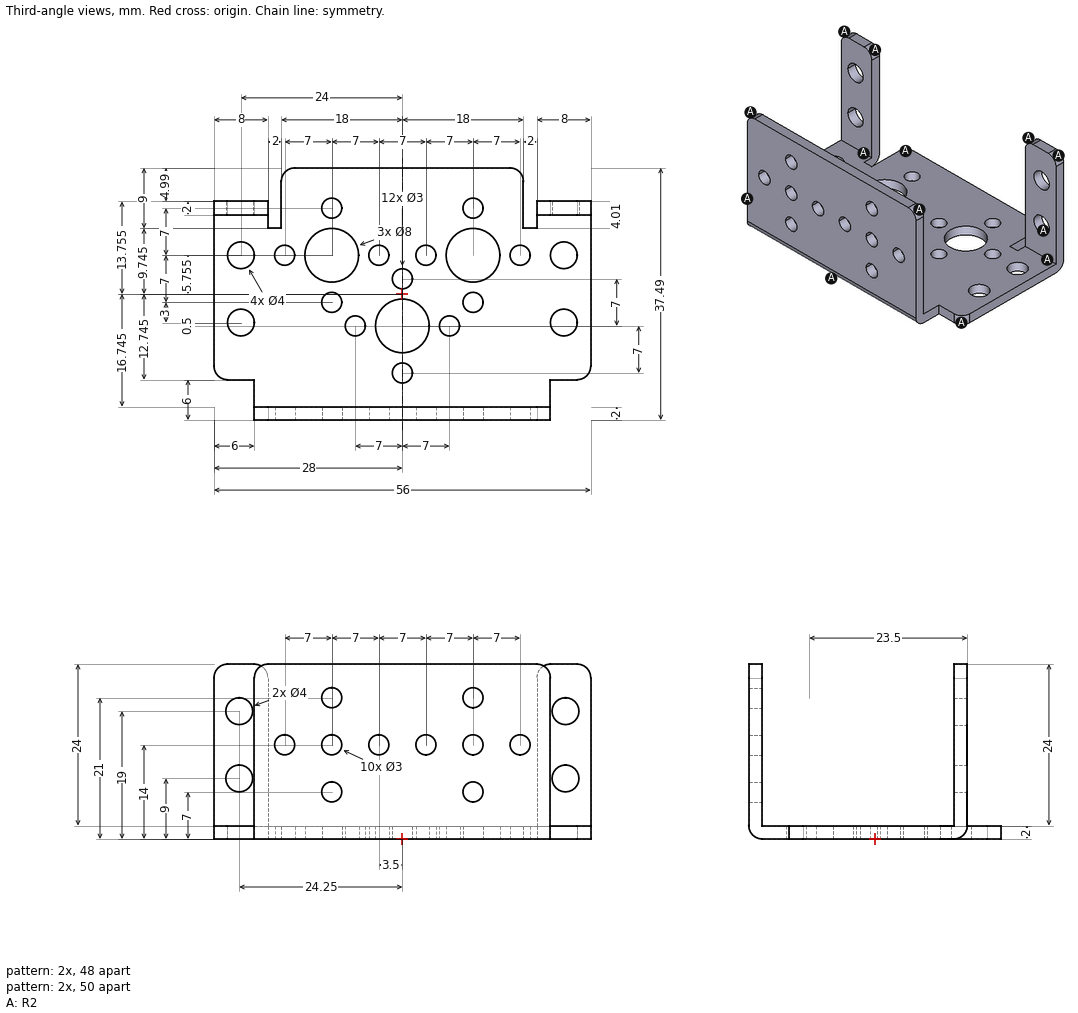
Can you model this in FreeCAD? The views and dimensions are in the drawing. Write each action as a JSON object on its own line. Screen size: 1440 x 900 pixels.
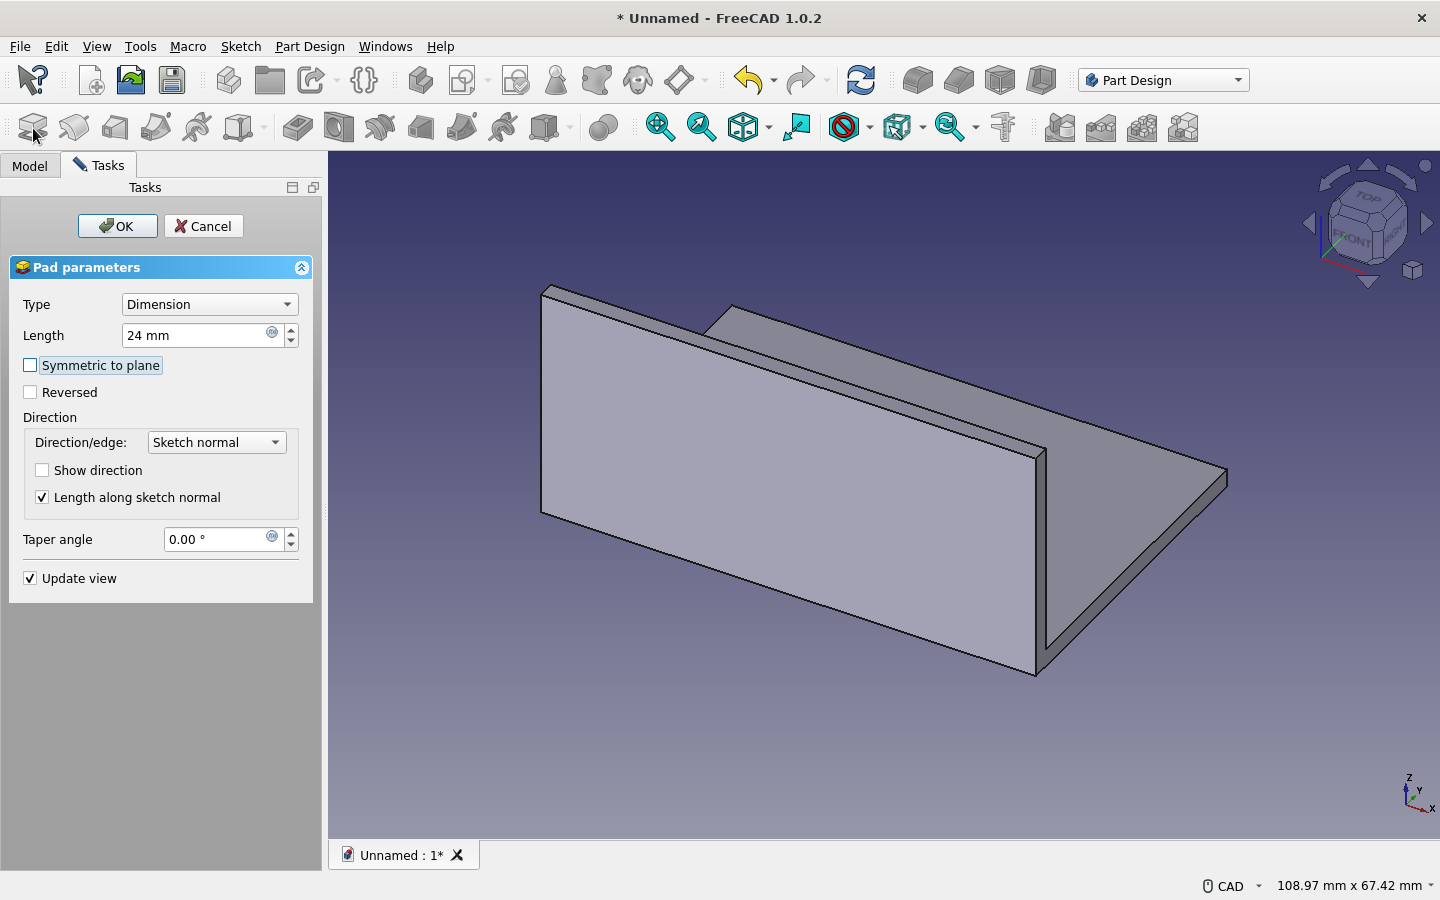
{"action": "left_click", "coordinate": [118, 226]}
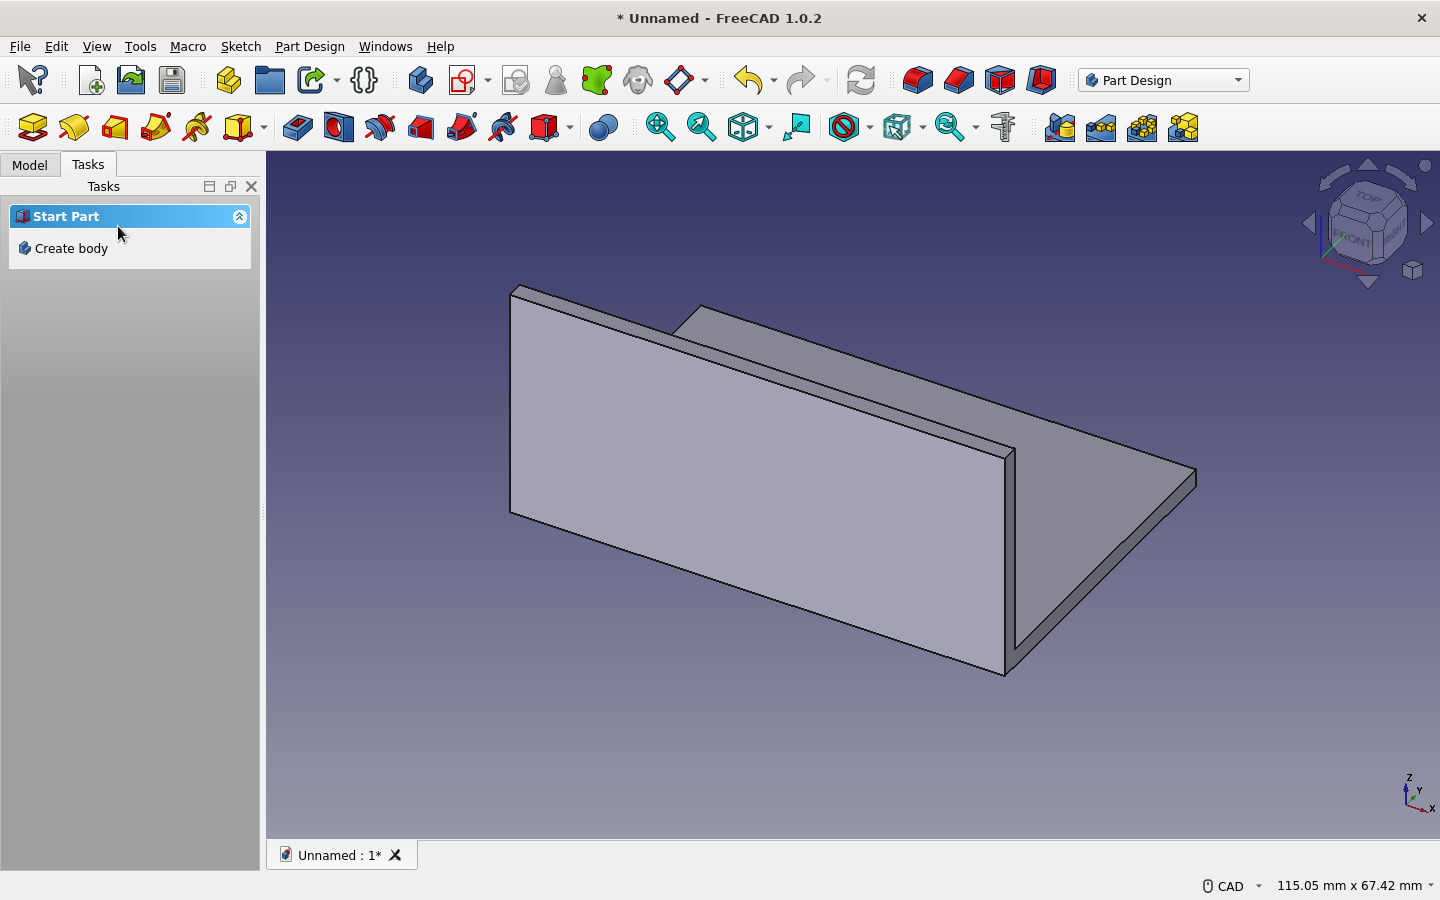
{"action": "key", "text": "v f"}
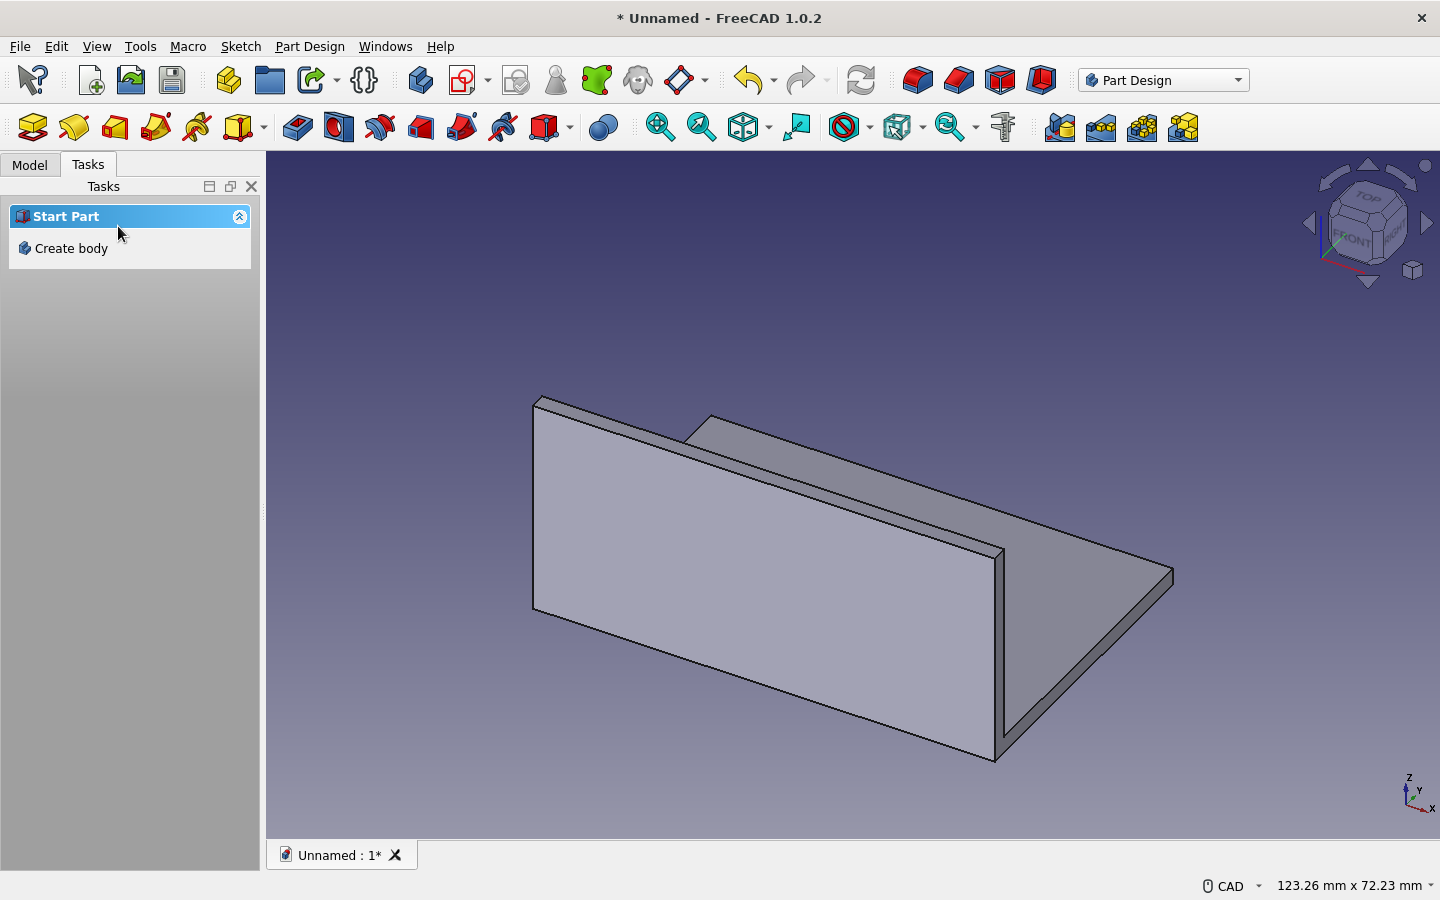
{"action": "key", "text": "0"}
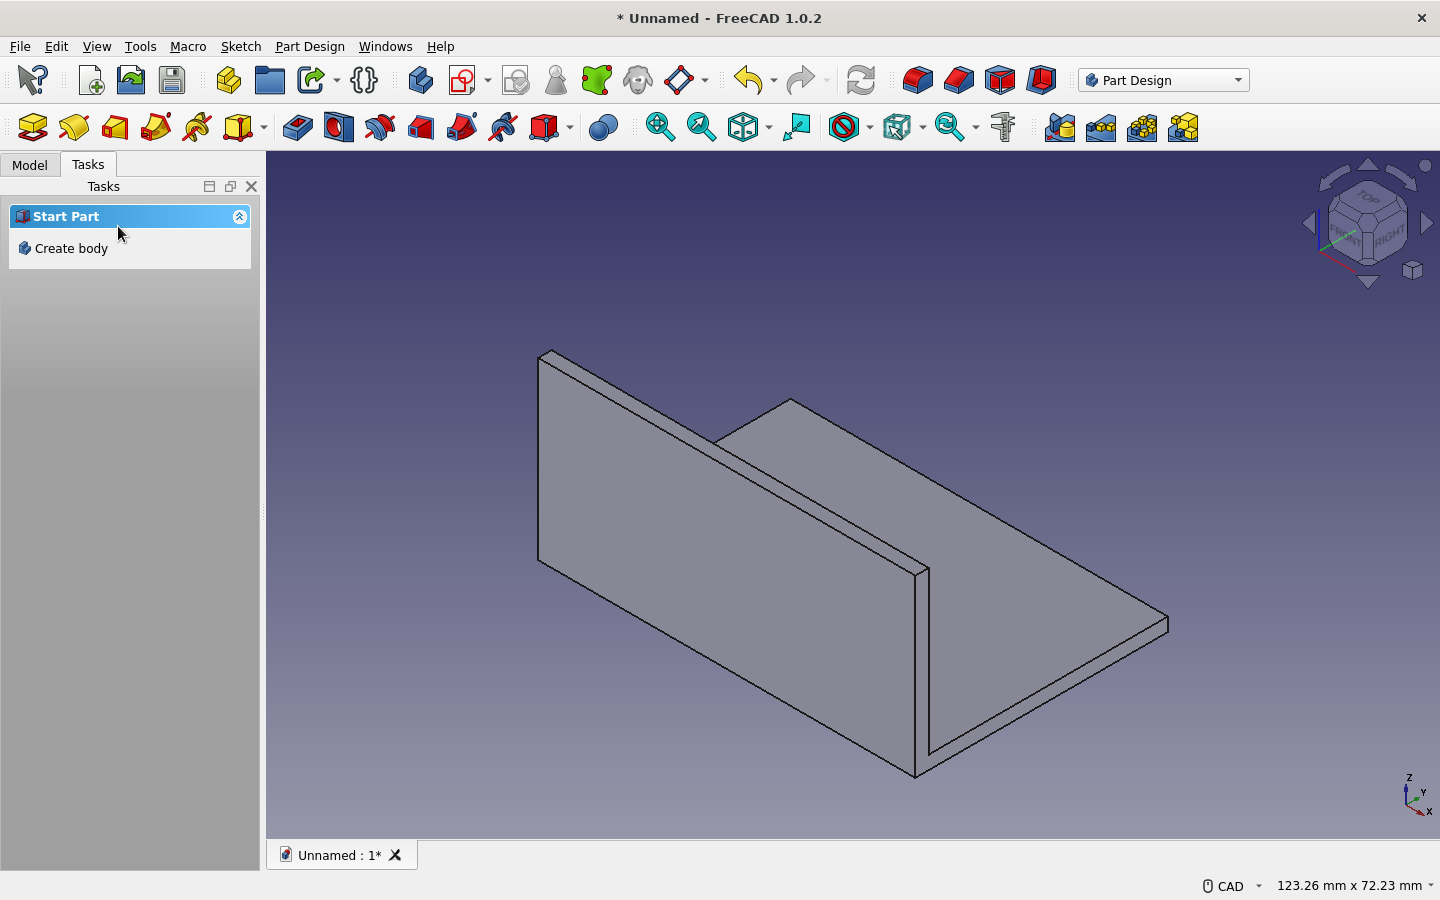
{"action": "left_click", "coordinate": [948, 587]}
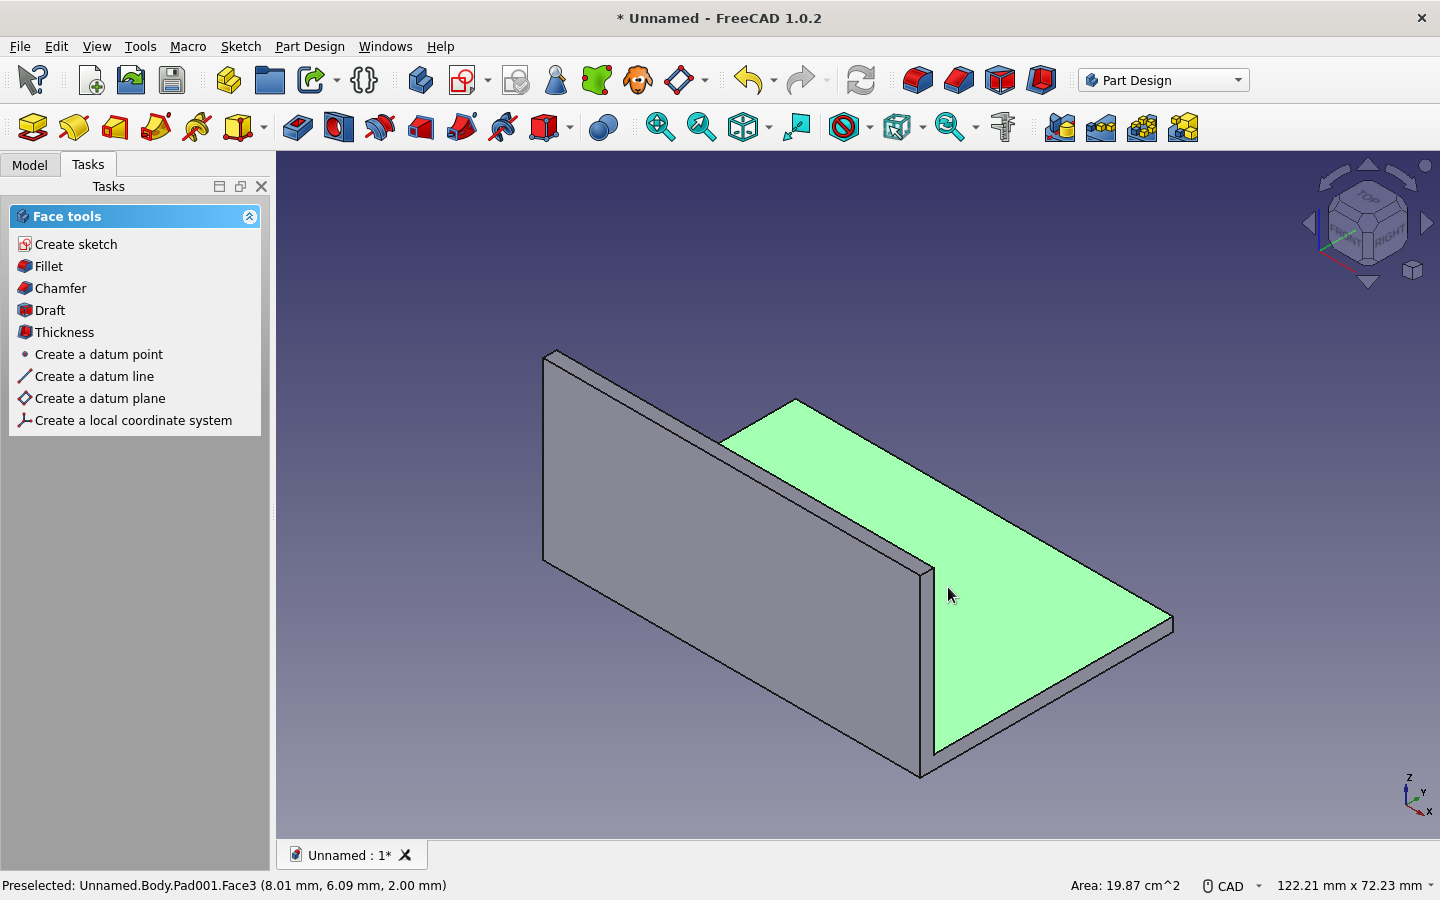
{"action": "left_click", "coordinate": [462, 80]}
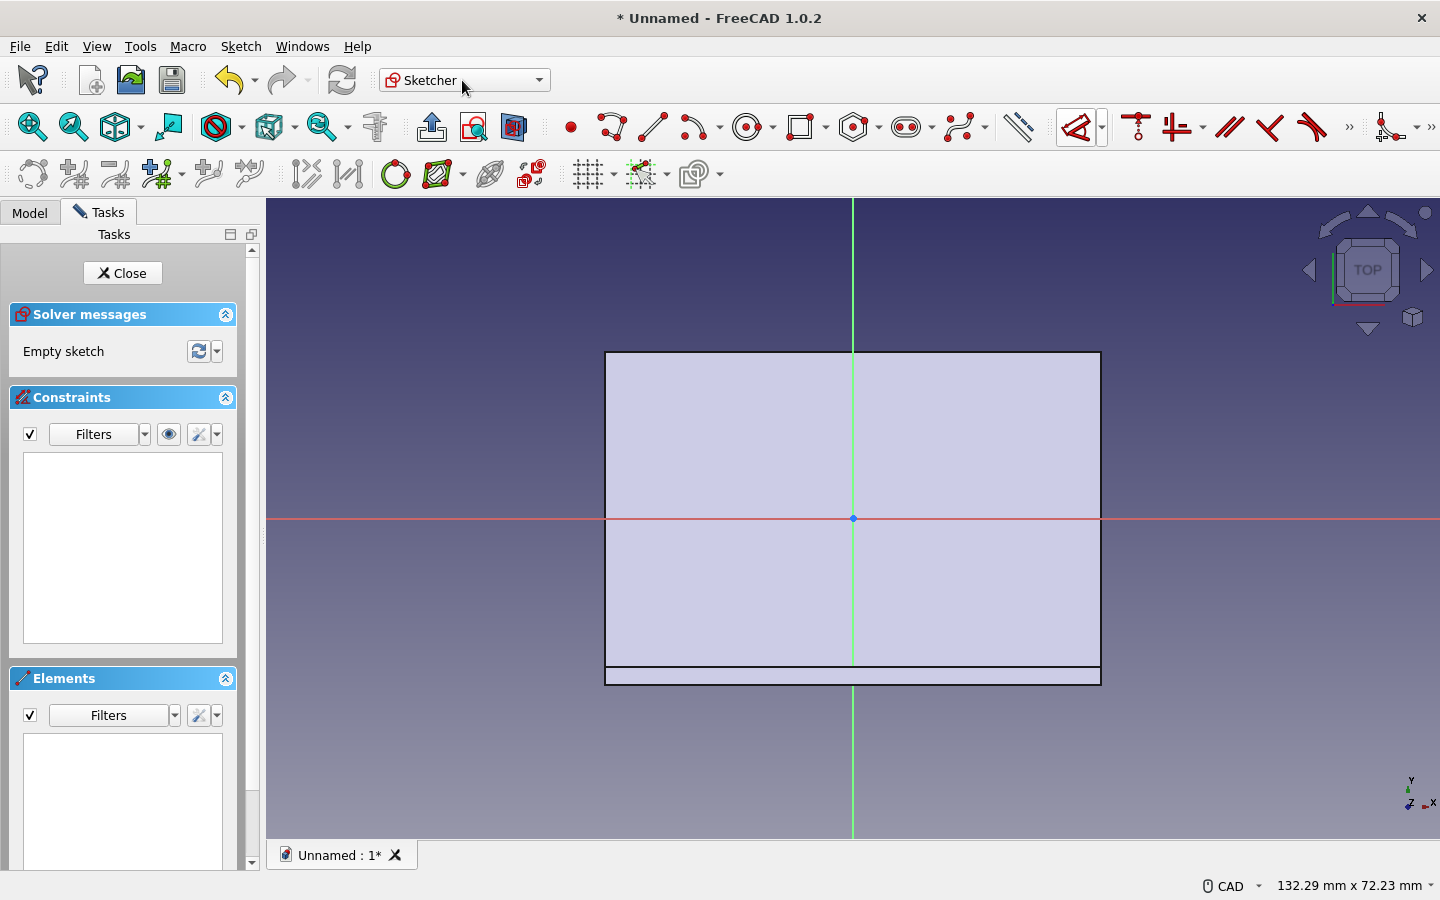
{"action": "scroll", "coordinate": [622, 391], "scroll_direction": "up", "scroll_amount": 11}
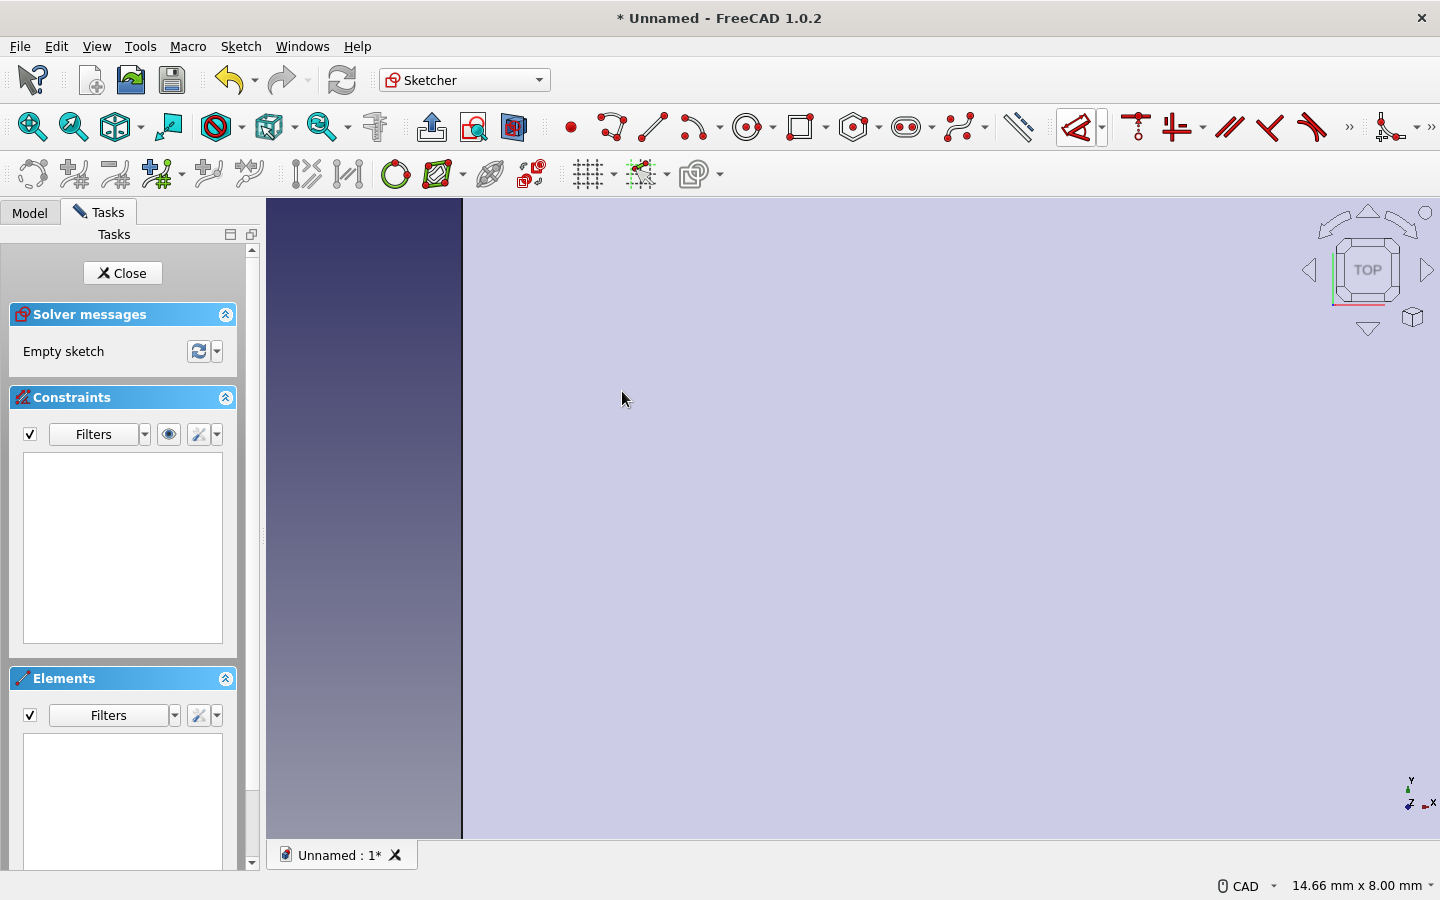
{"action": "left_click", "coordinate": [800, 128]}